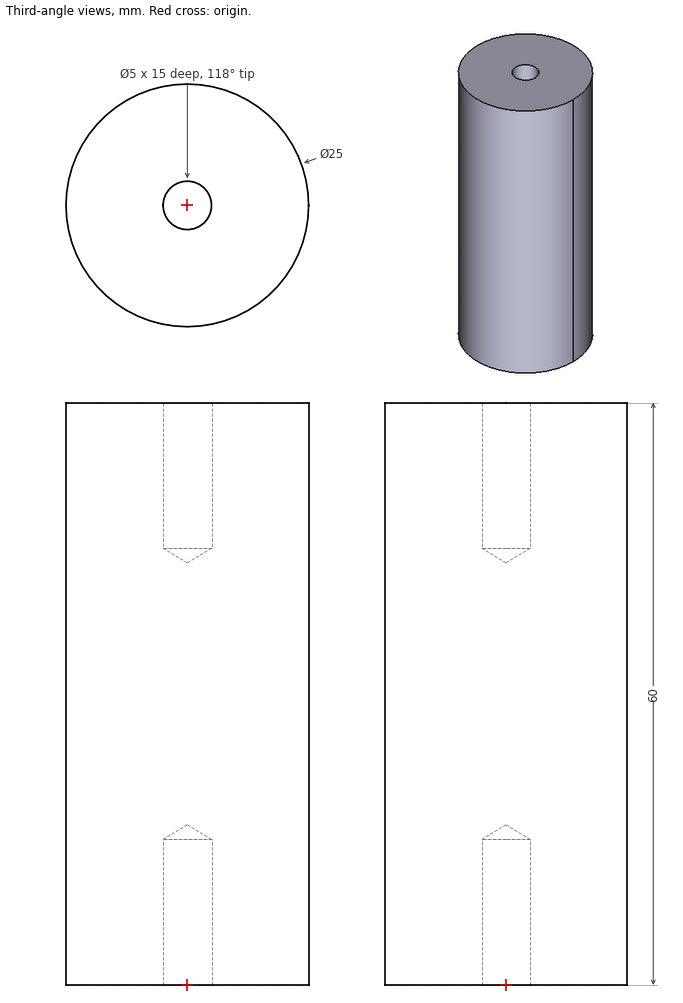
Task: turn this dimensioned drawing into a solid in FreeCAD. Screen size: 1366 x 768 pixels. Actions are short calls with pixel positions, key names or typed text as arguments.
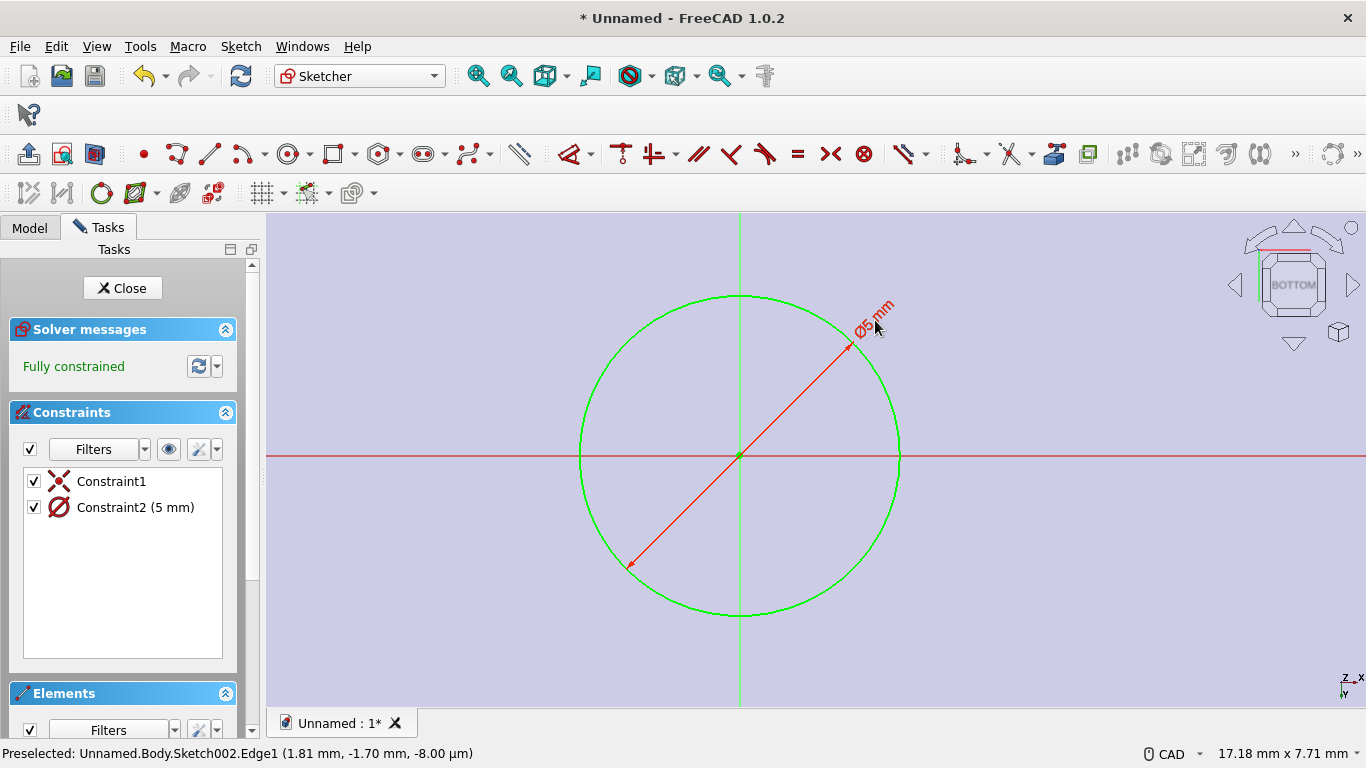
click(123, 288)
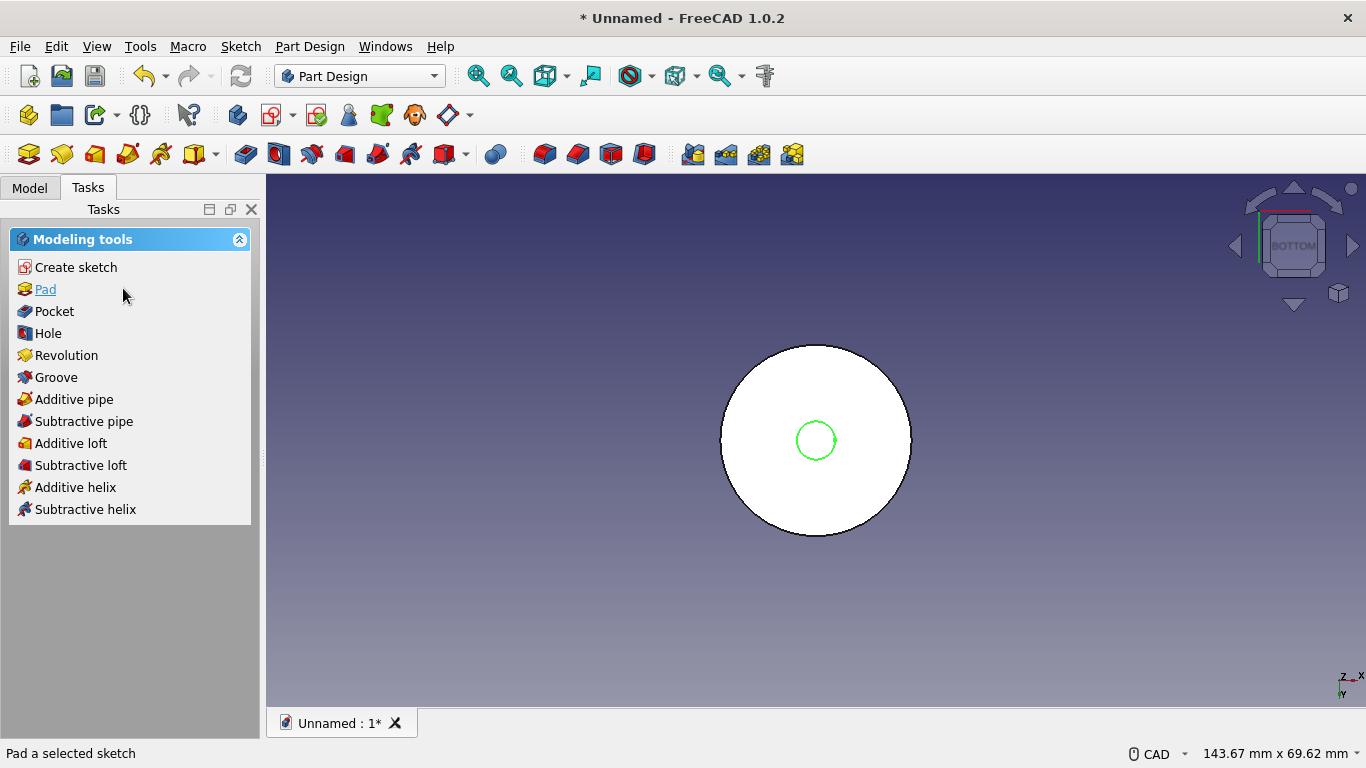
click(279, 154)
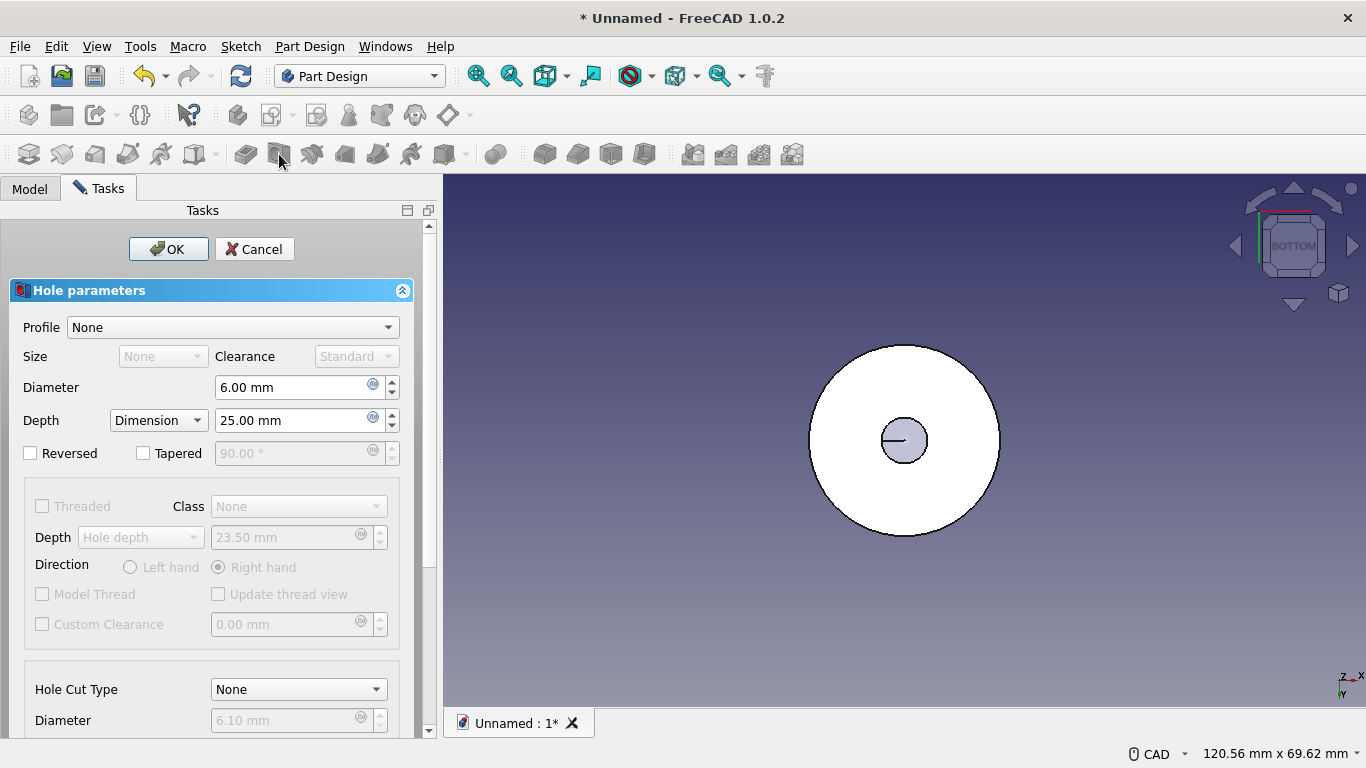
triple_click(300, 388)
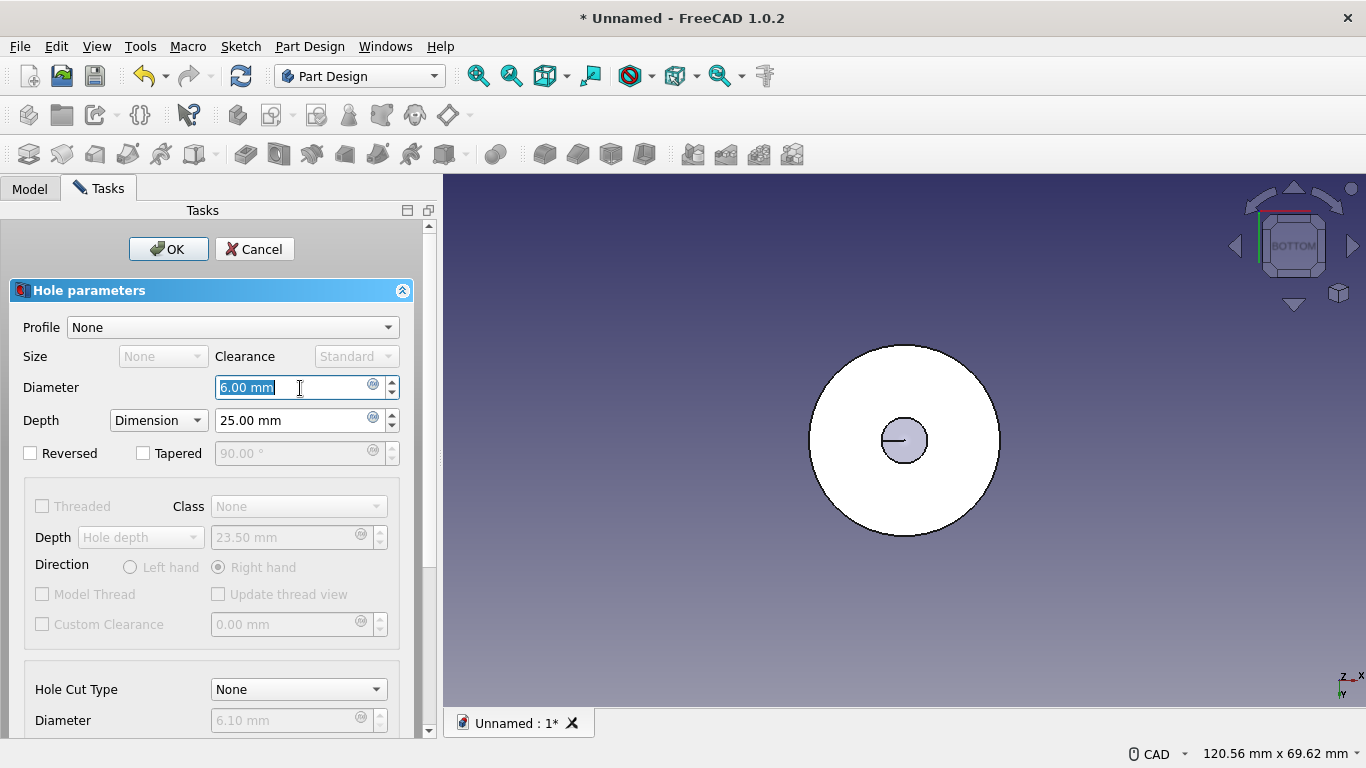
text(5)
key(Tab)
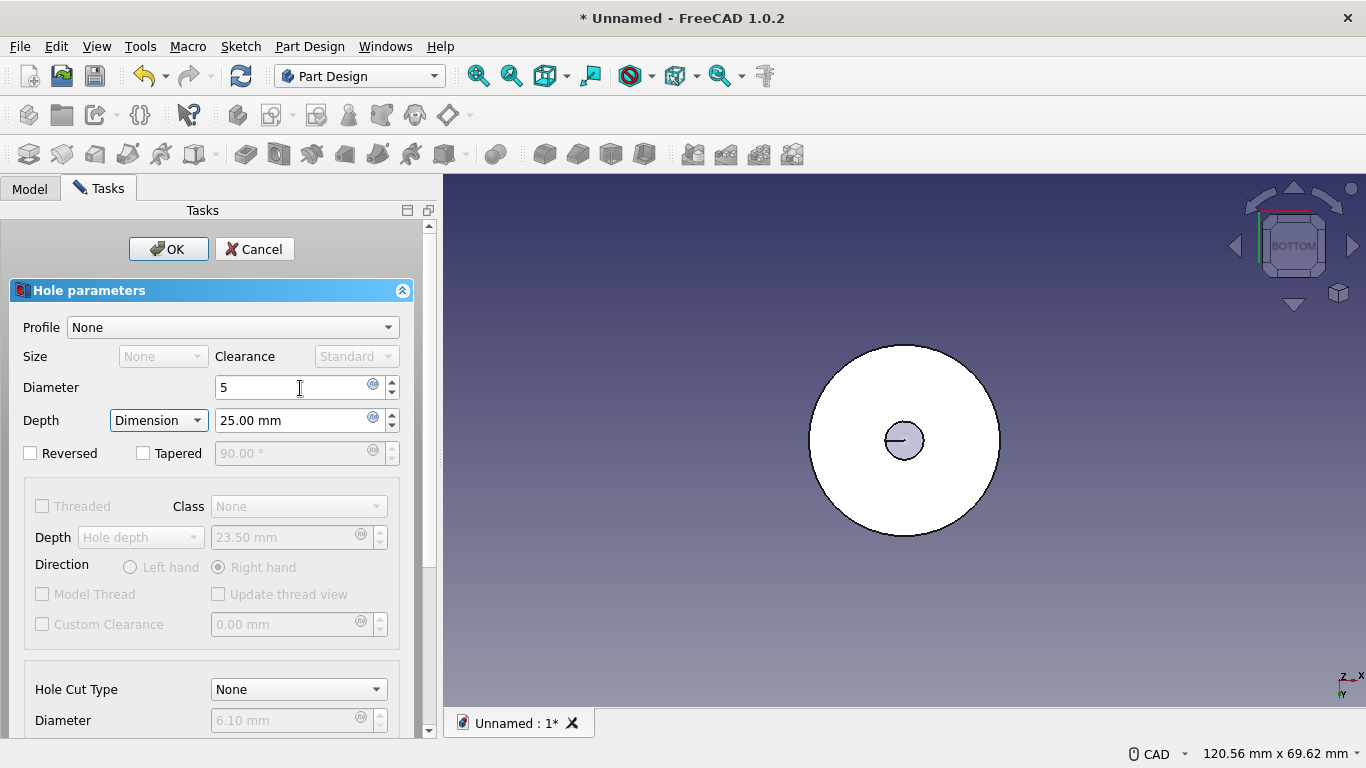
triple_click(300, 420)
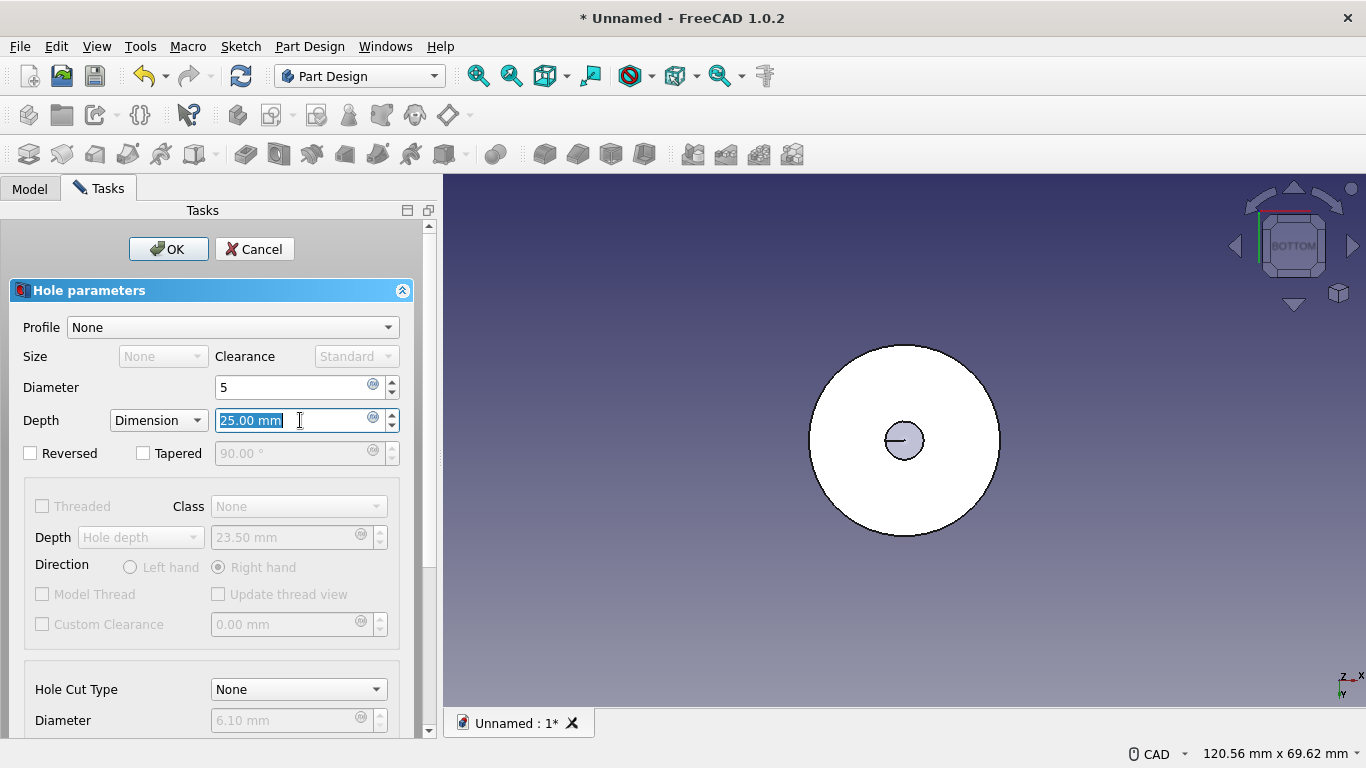
text(15)
key(Tab)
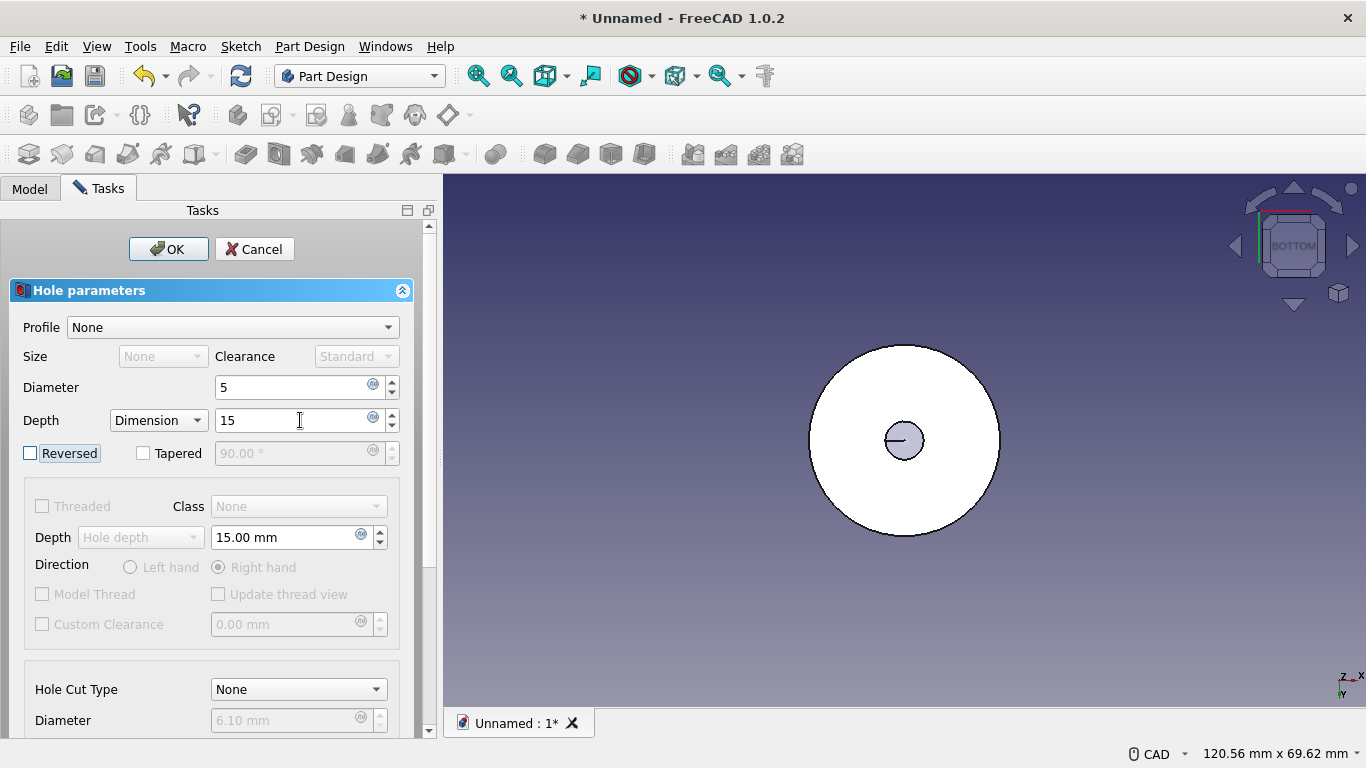
click(169, 249)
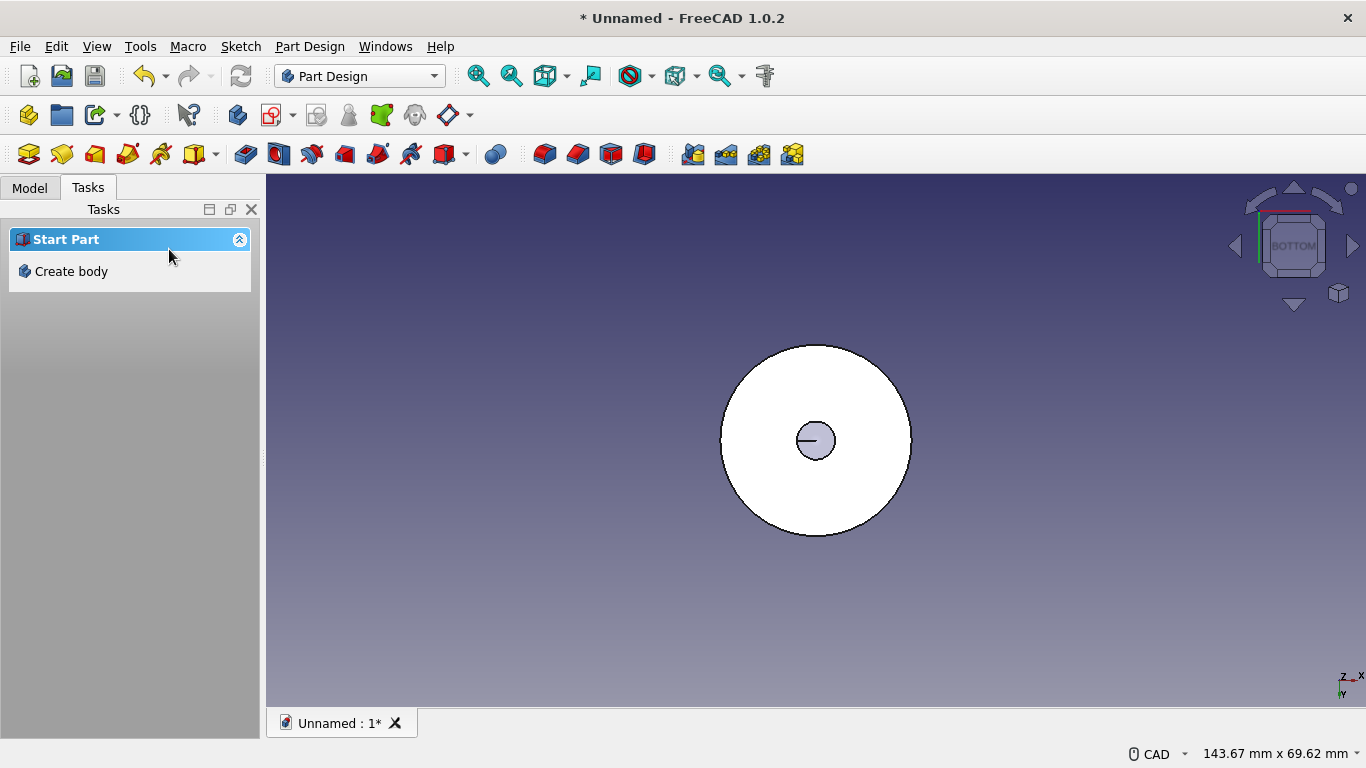
key(0)